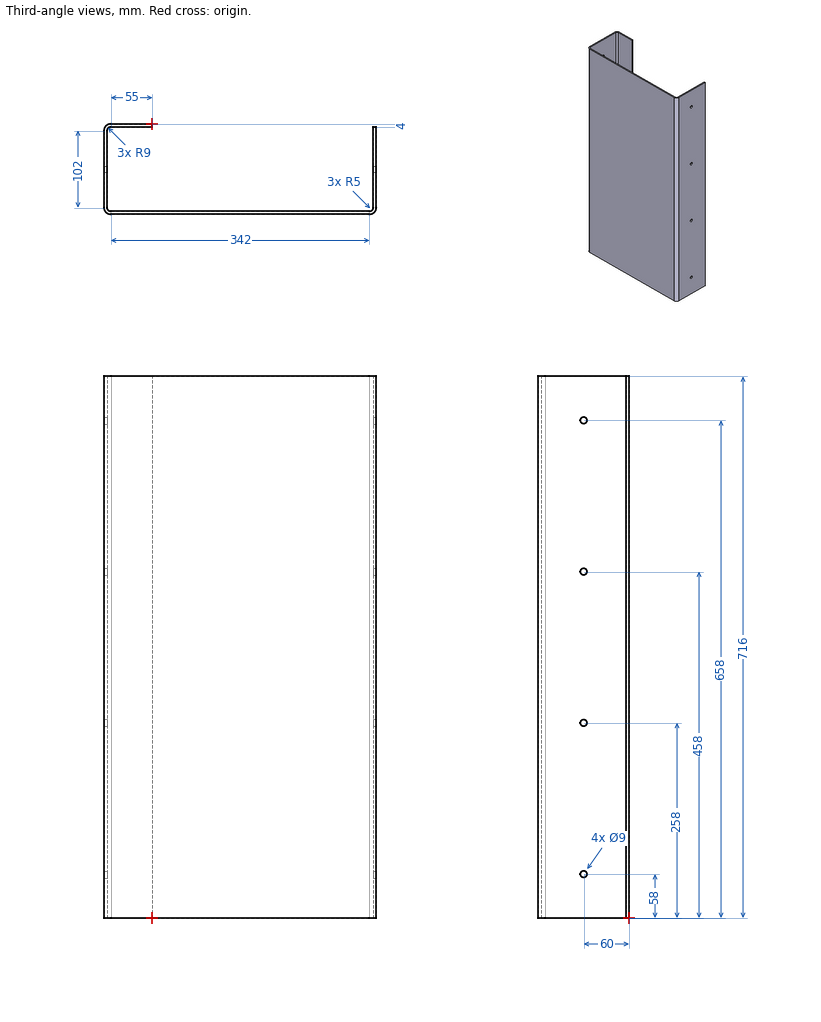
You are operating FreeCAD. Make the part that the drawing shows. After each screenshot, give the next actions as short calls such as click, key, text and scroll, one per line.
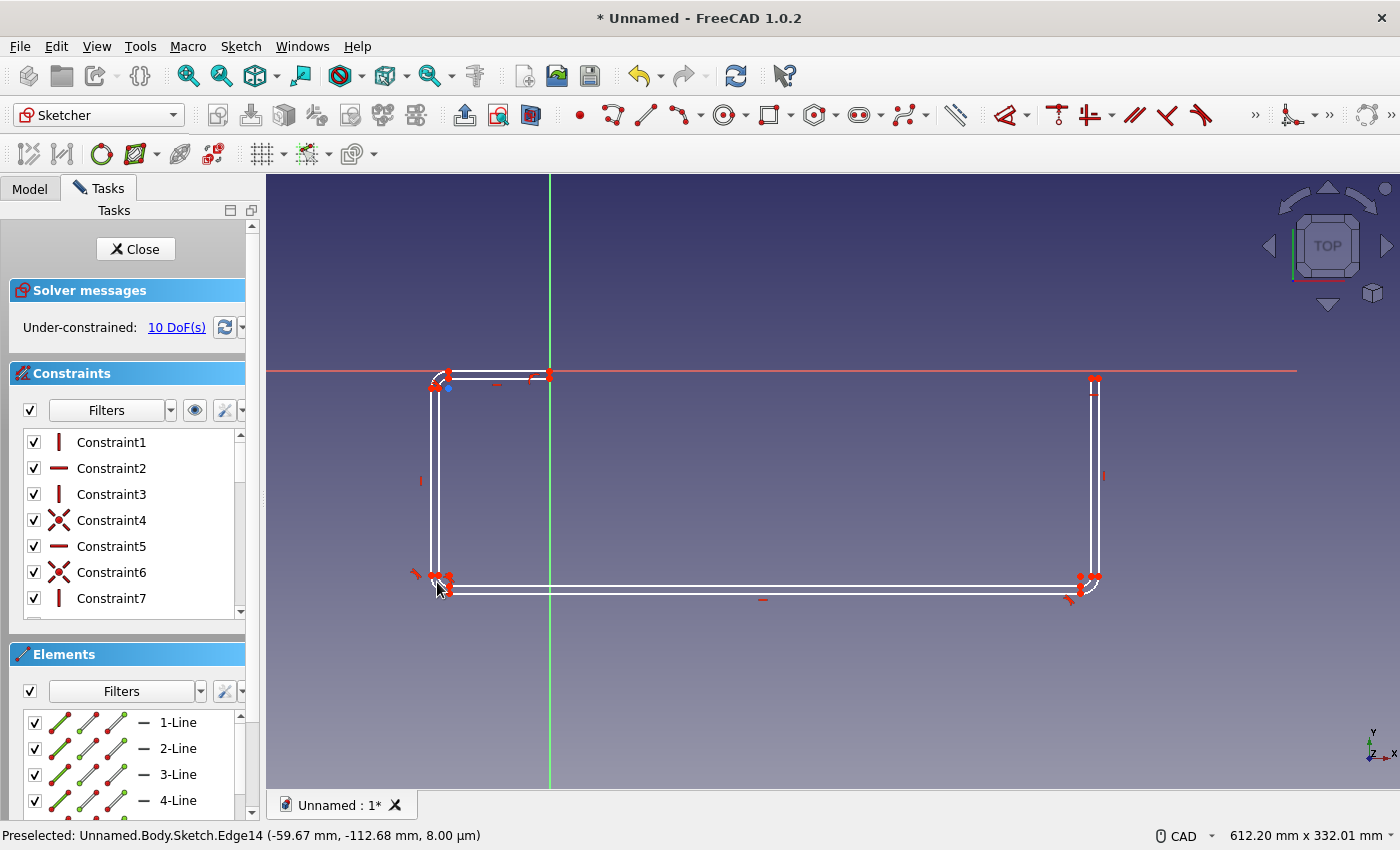
scroll(444, 380, up, 6)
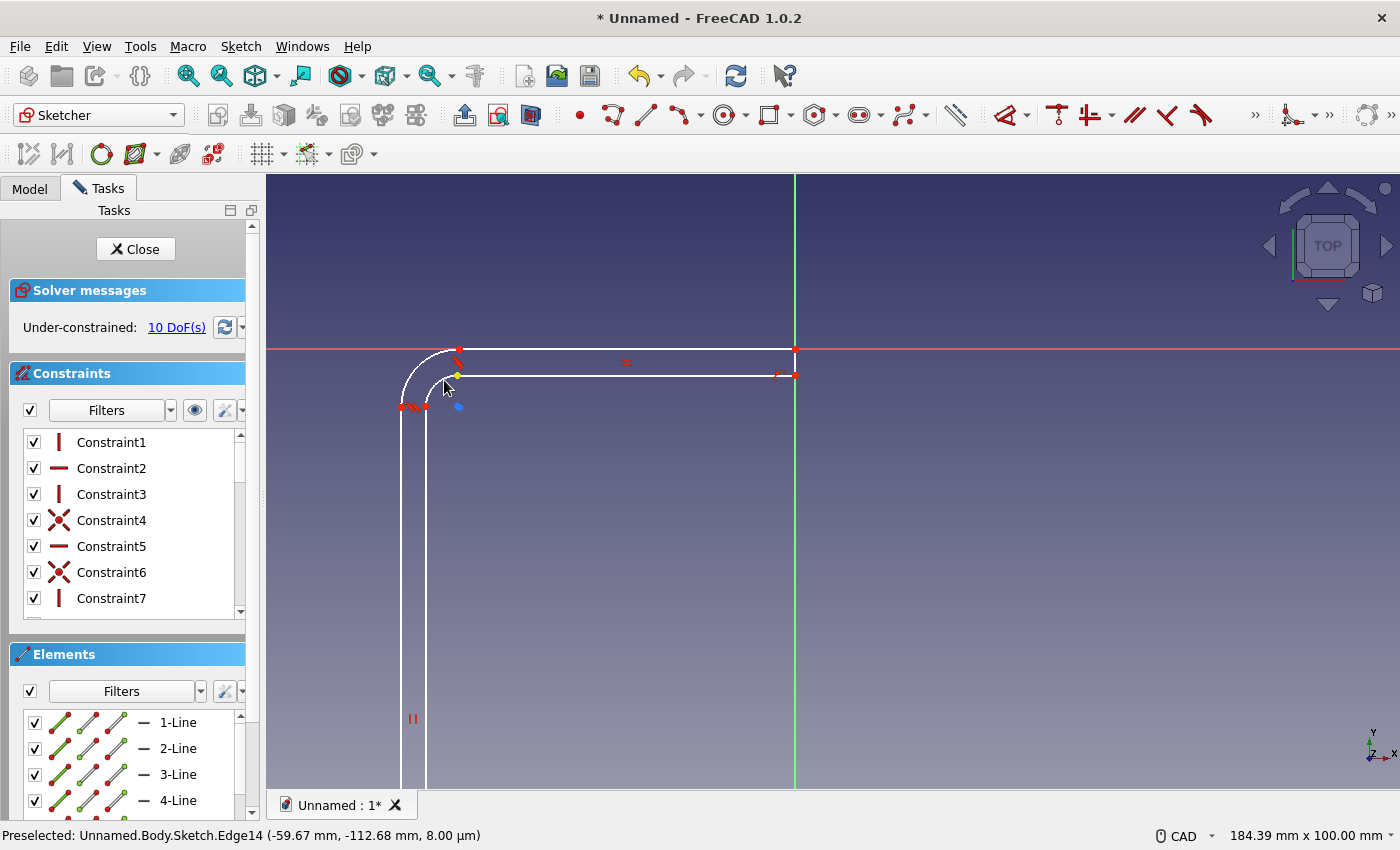
click(443, 379)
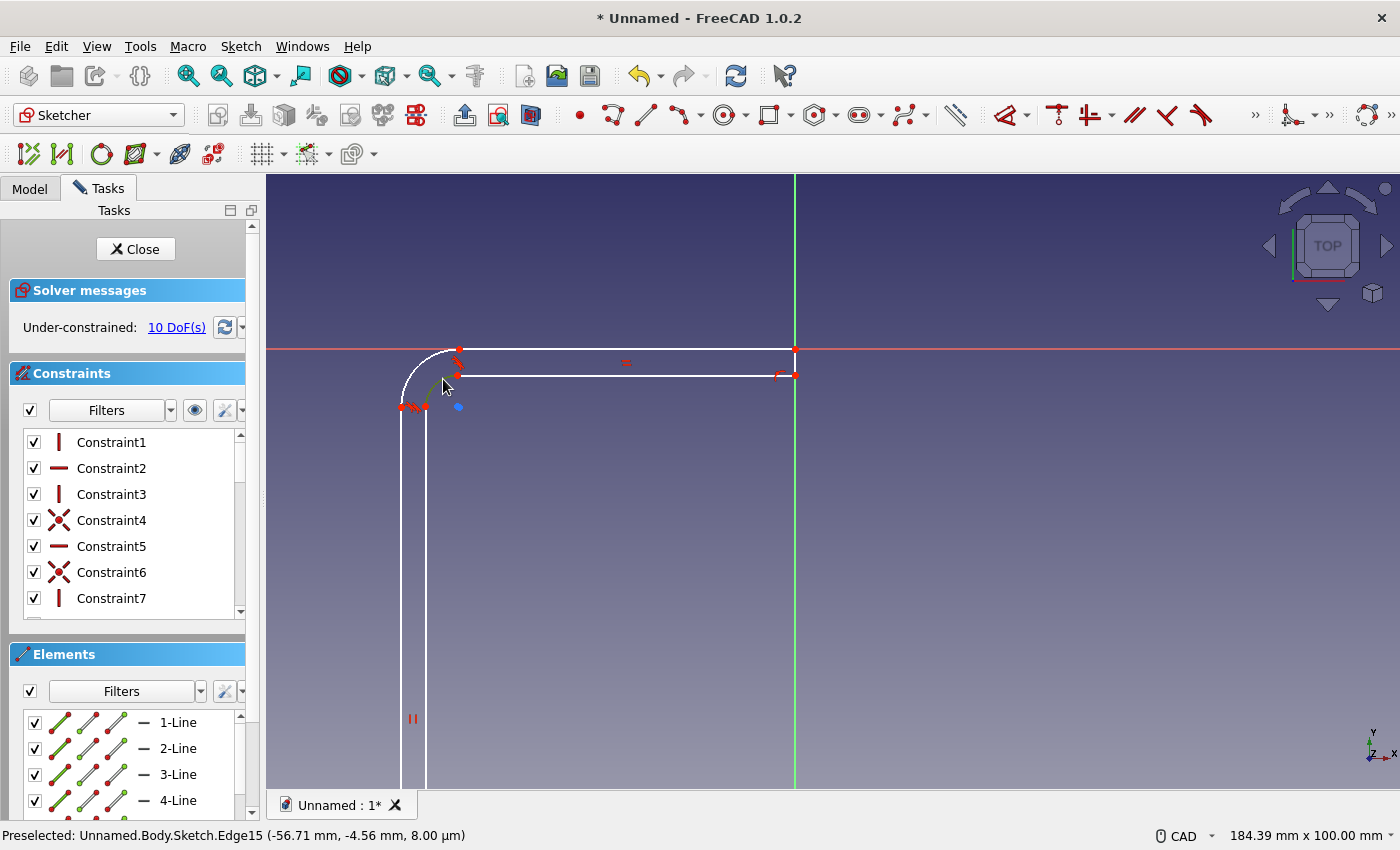
click(408, 381)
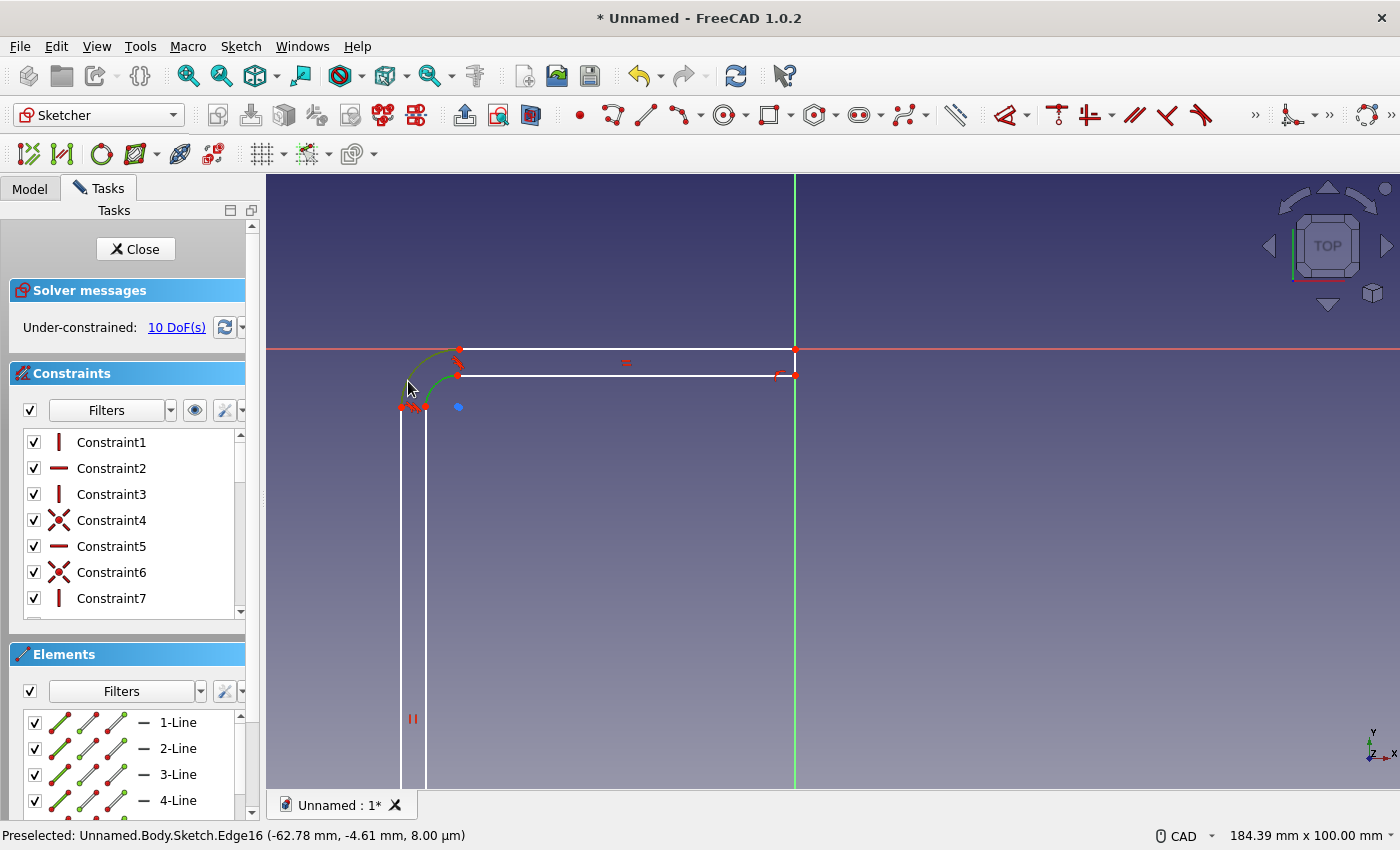
click(1057, 116)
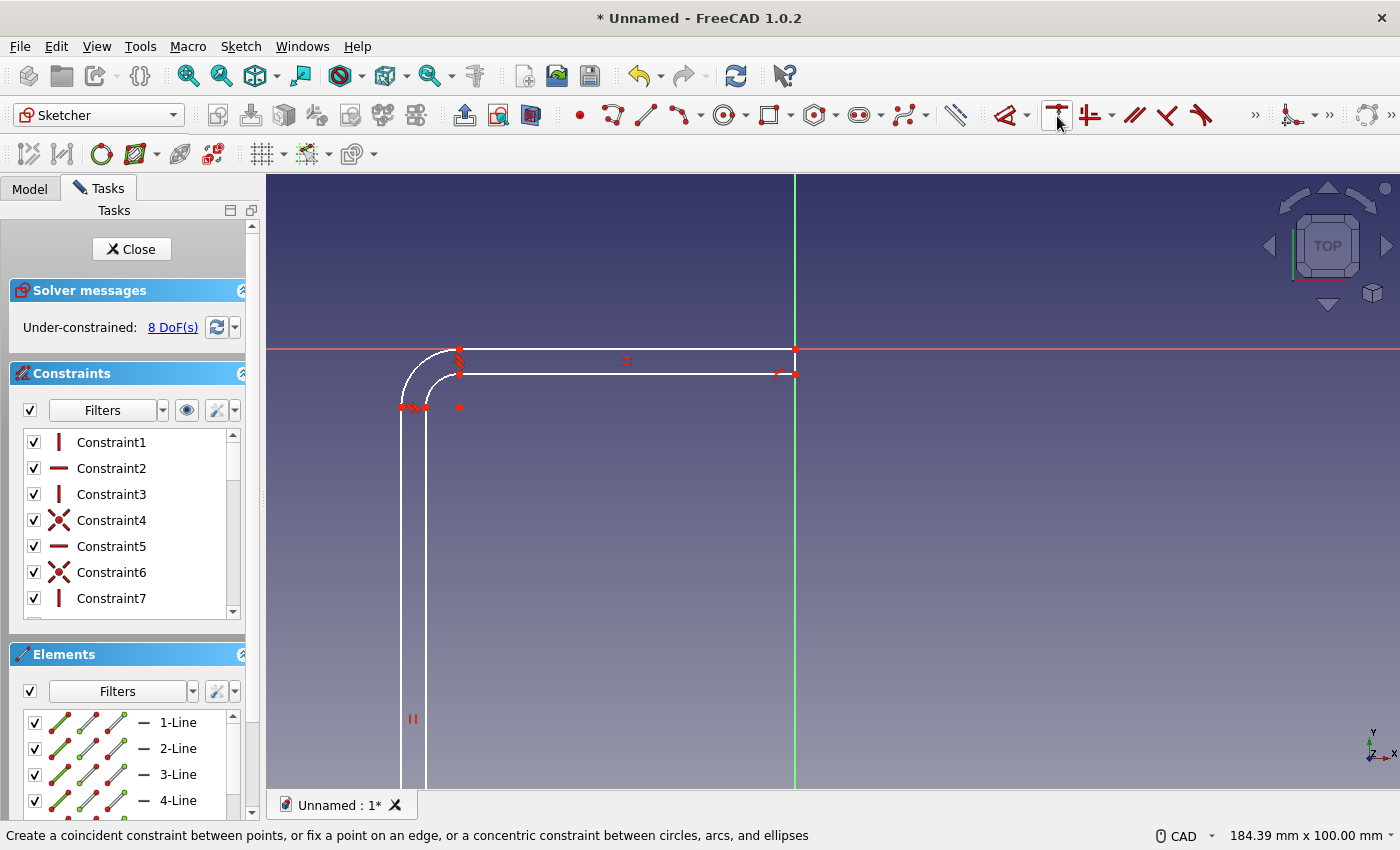
scroll(444, 379, down, 6)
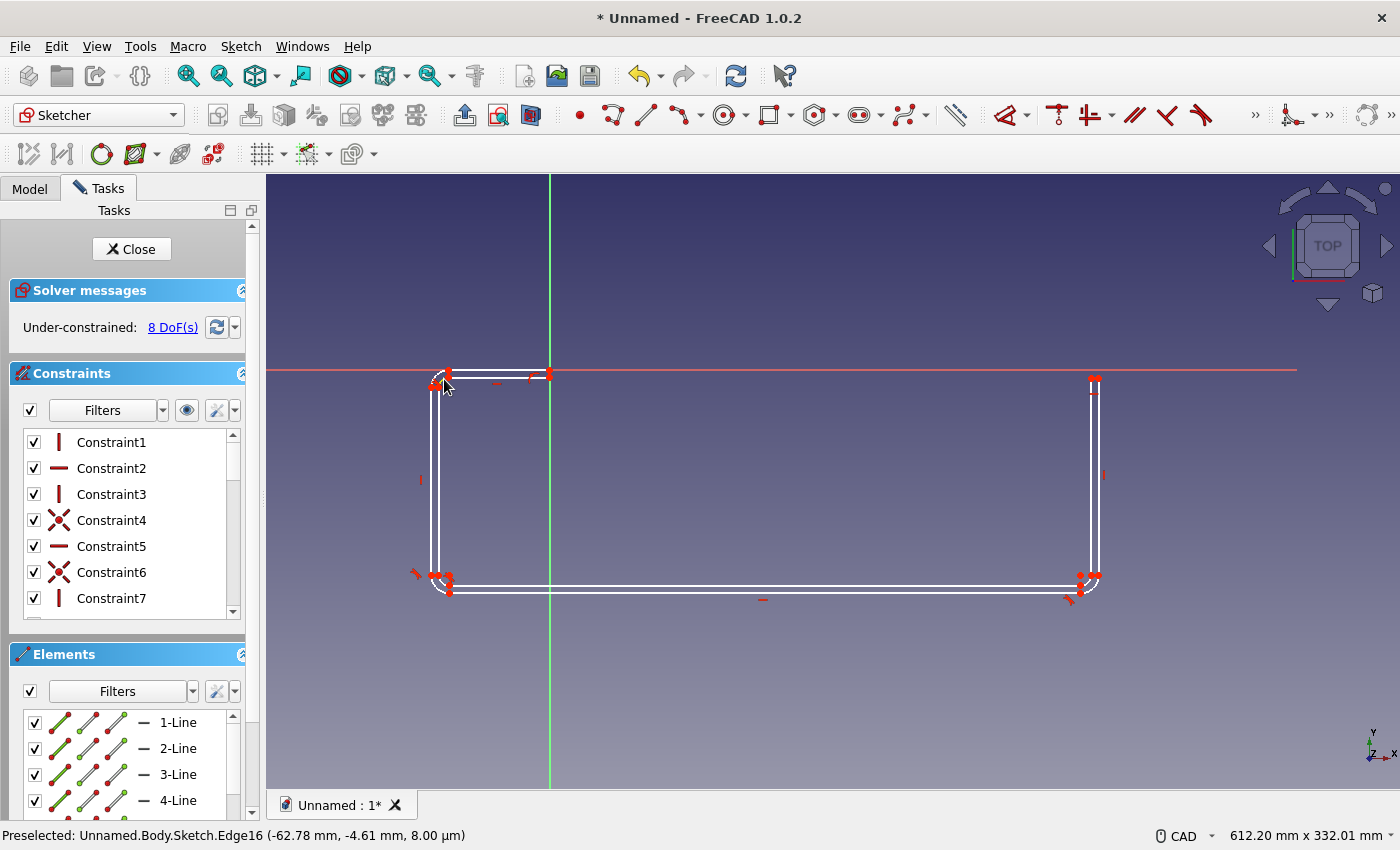
scroll(433, 583, up, 4)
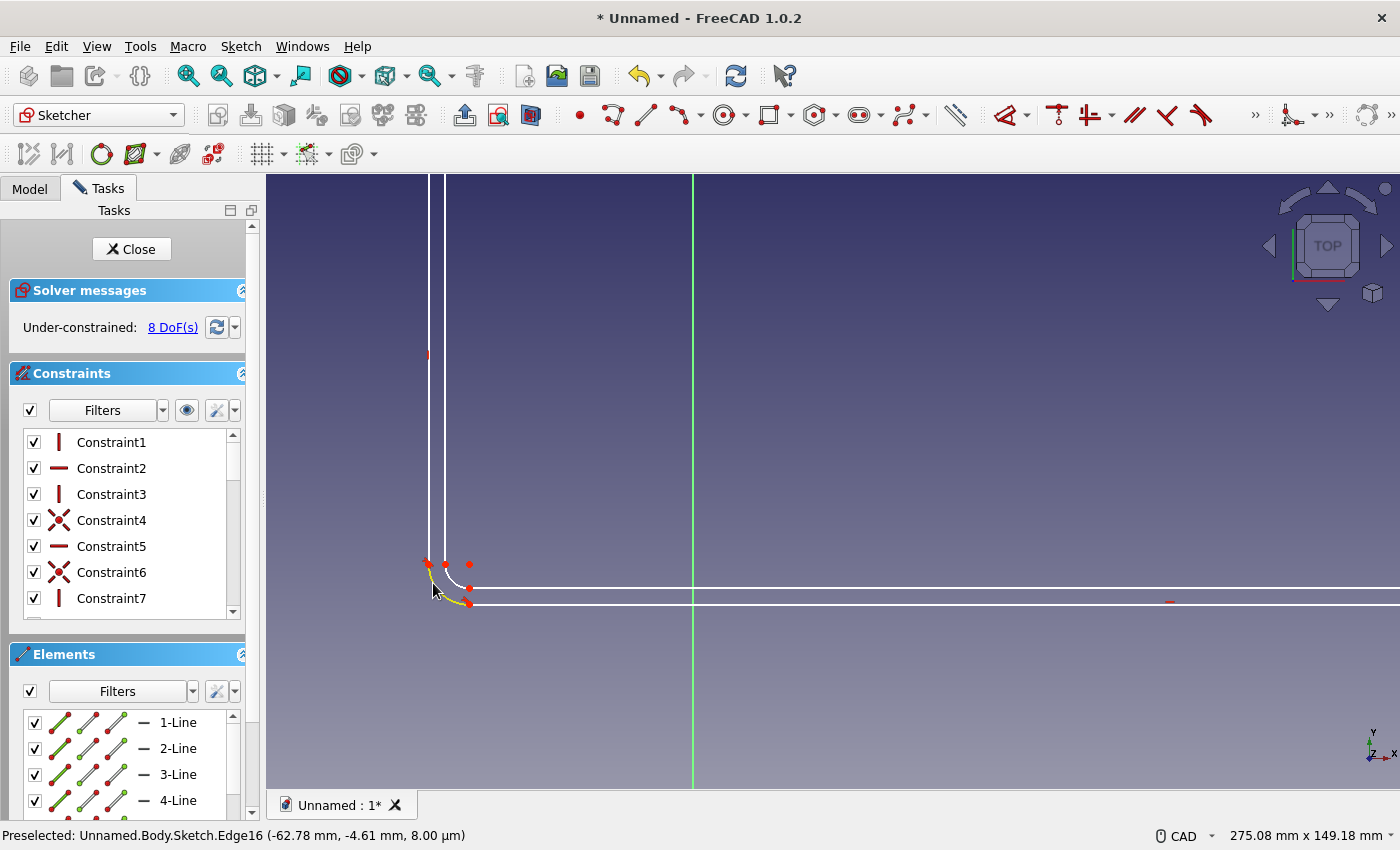
click(433, 583)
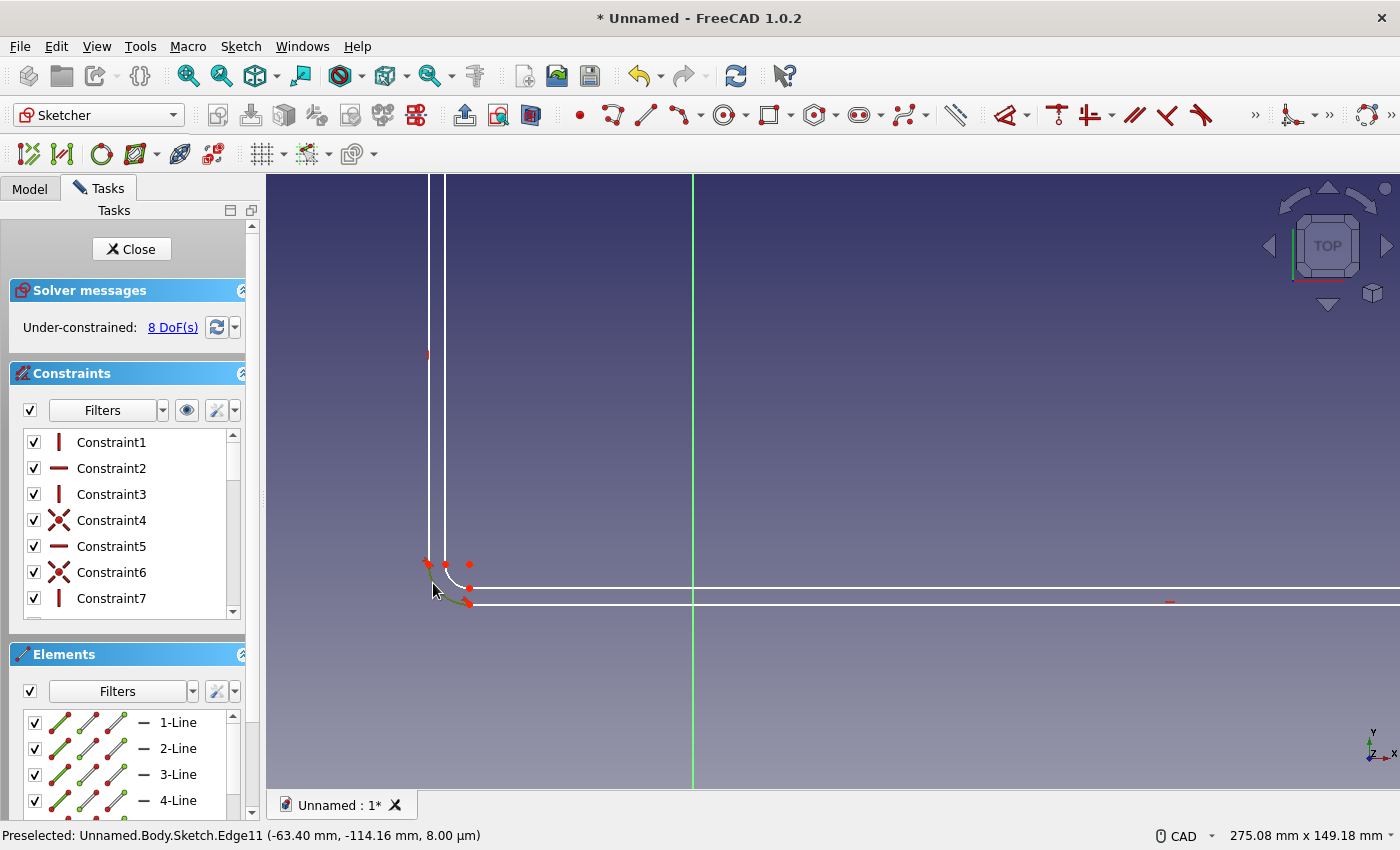
scroll(433, 584, down, 4)